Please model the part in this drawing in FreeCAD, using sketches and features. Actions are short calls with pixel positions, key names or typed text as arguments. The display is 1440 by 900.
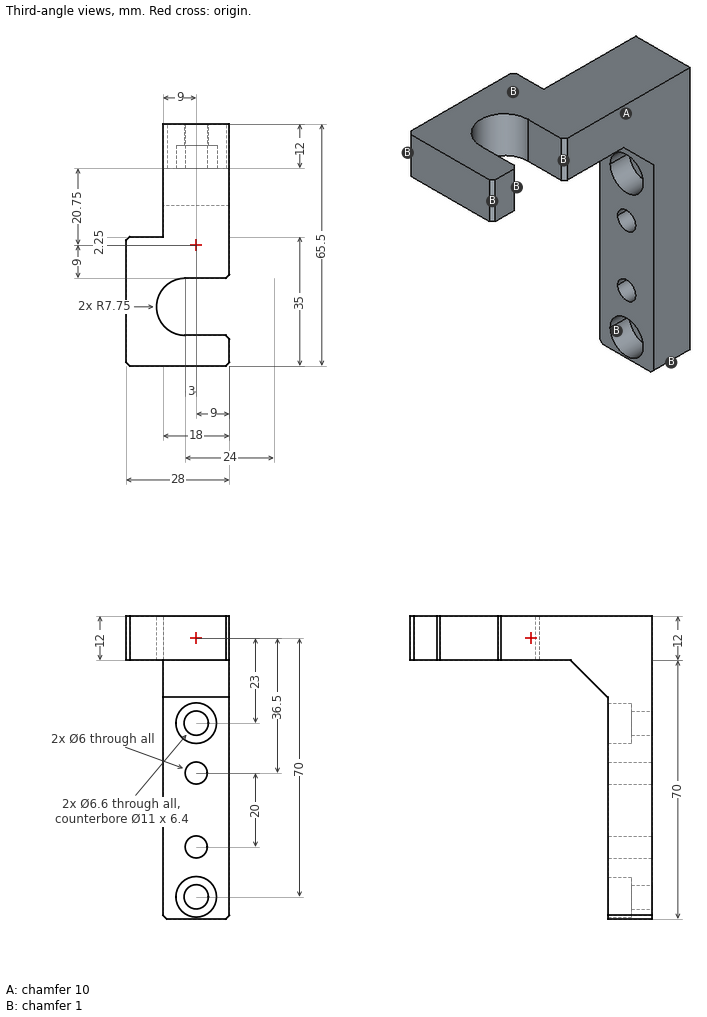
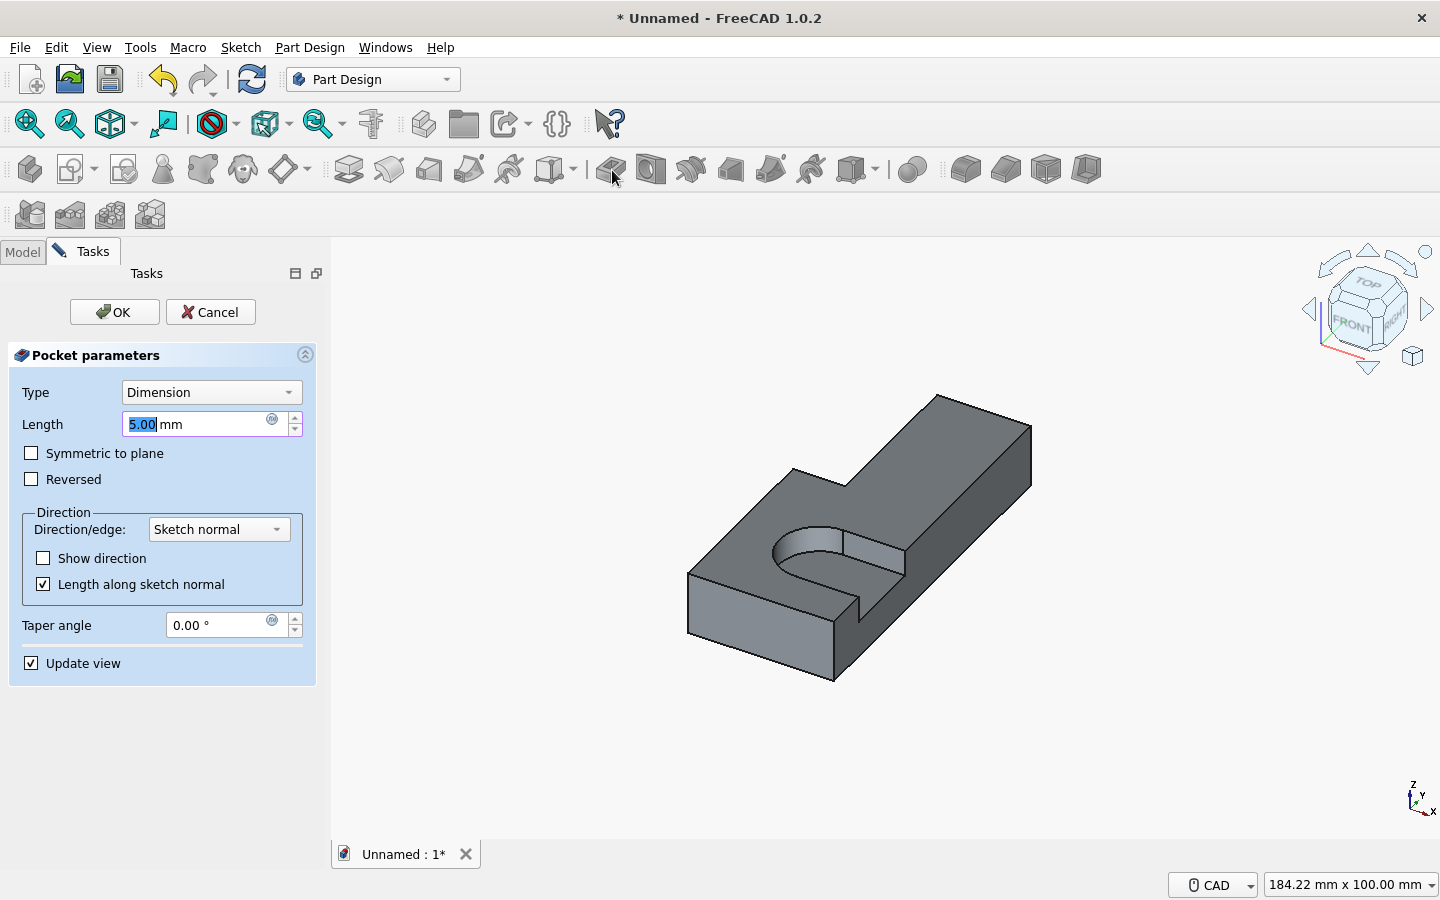
click(212, 392)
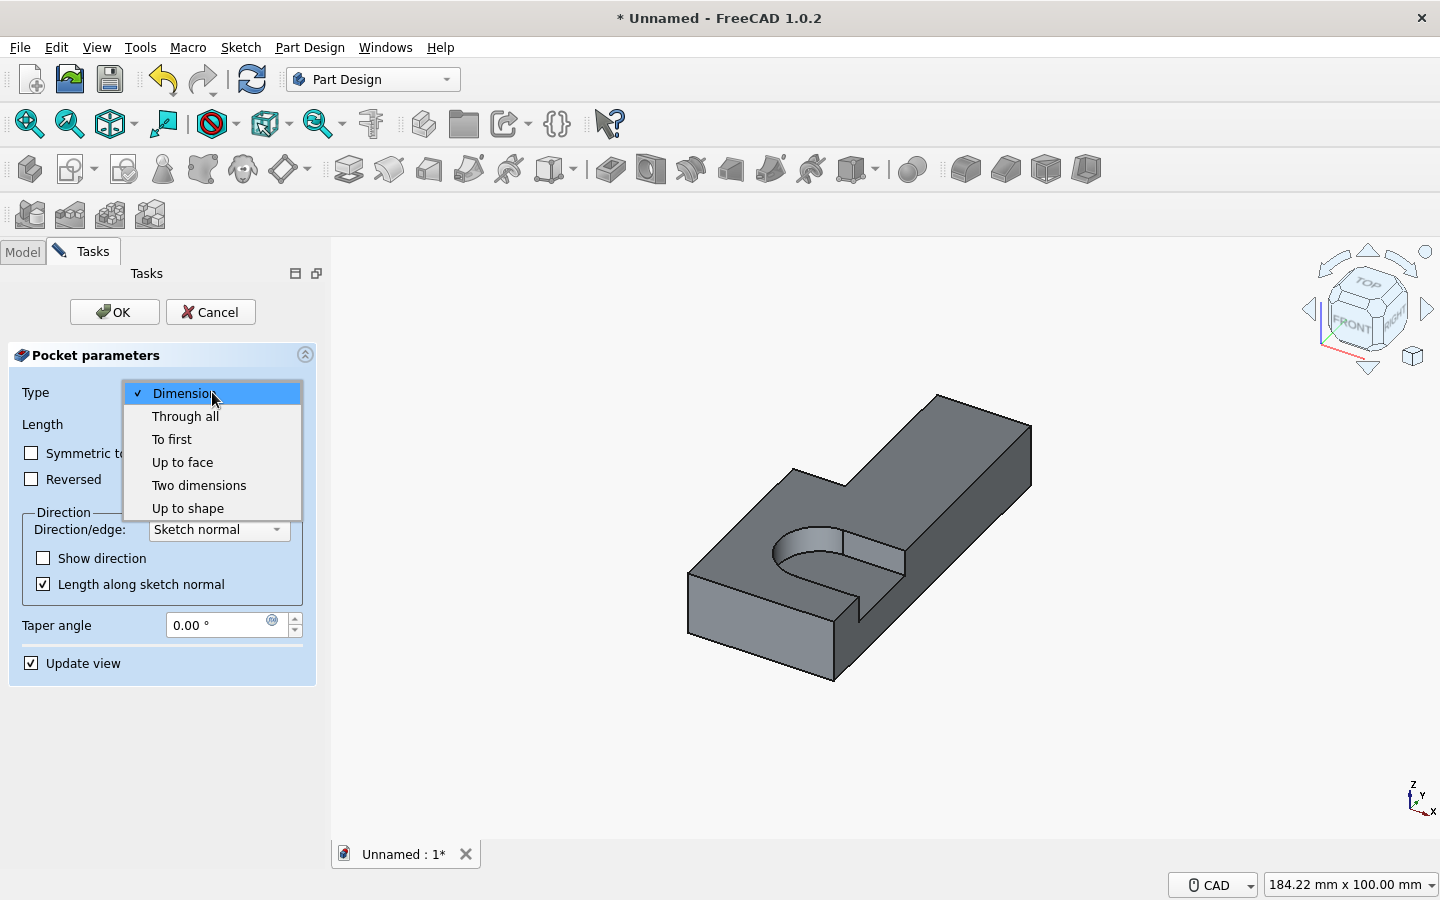
click(212, 416)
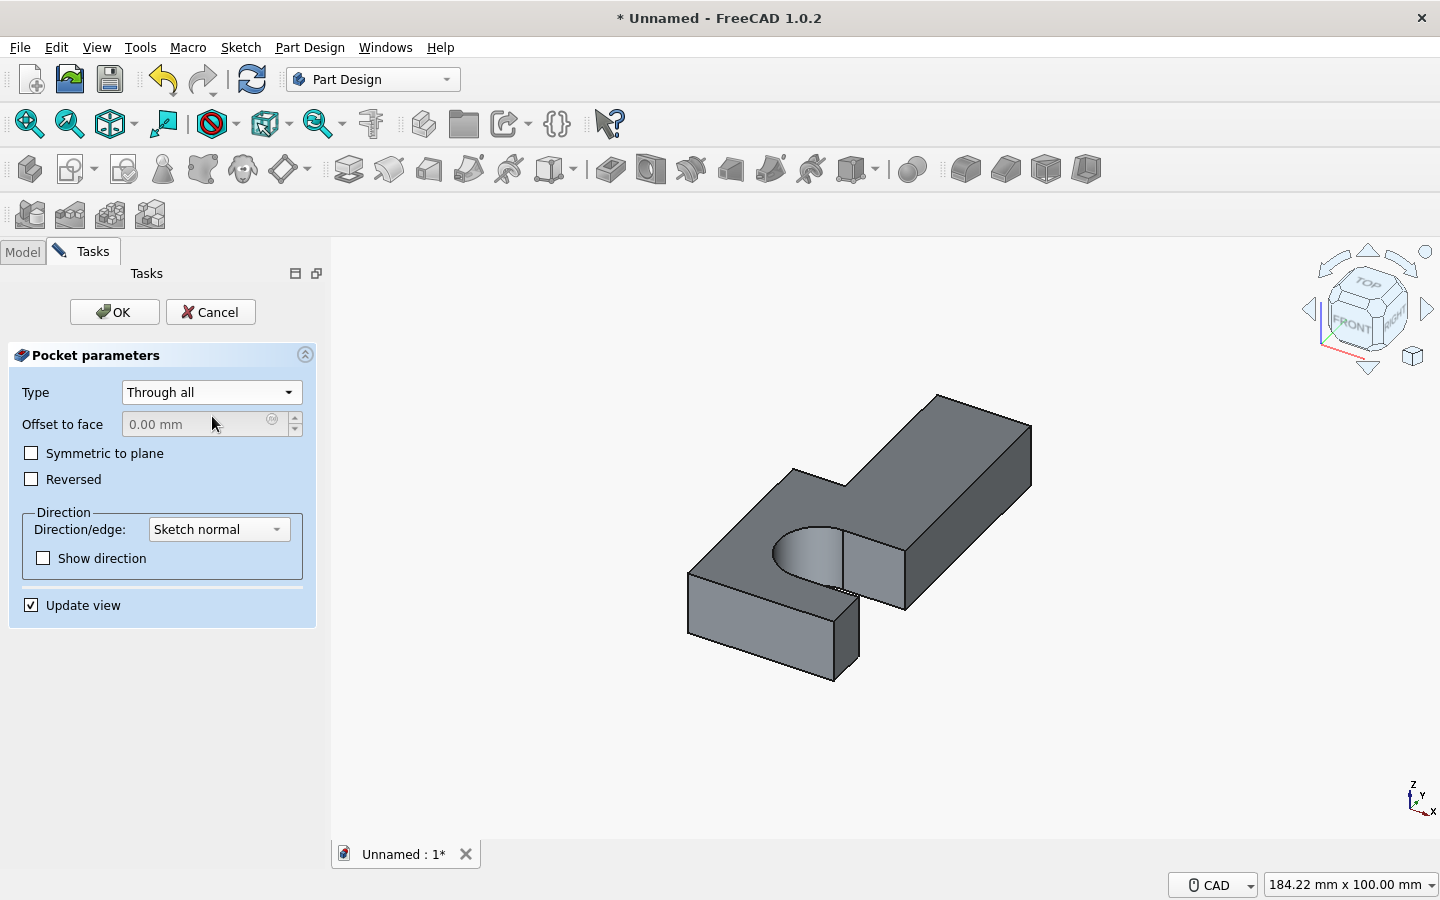
click(115, 312)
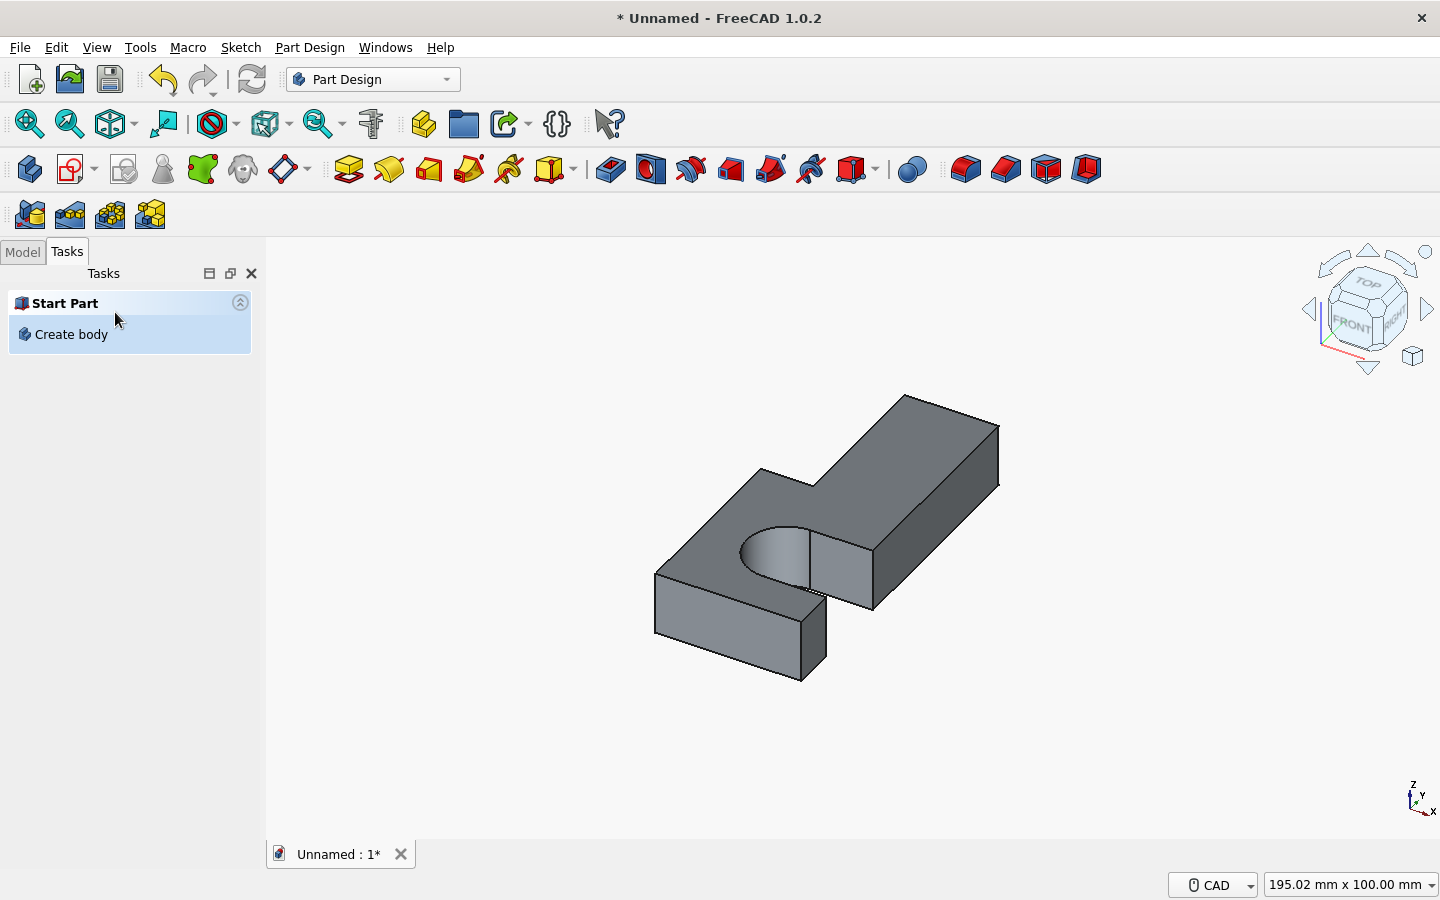
key(5)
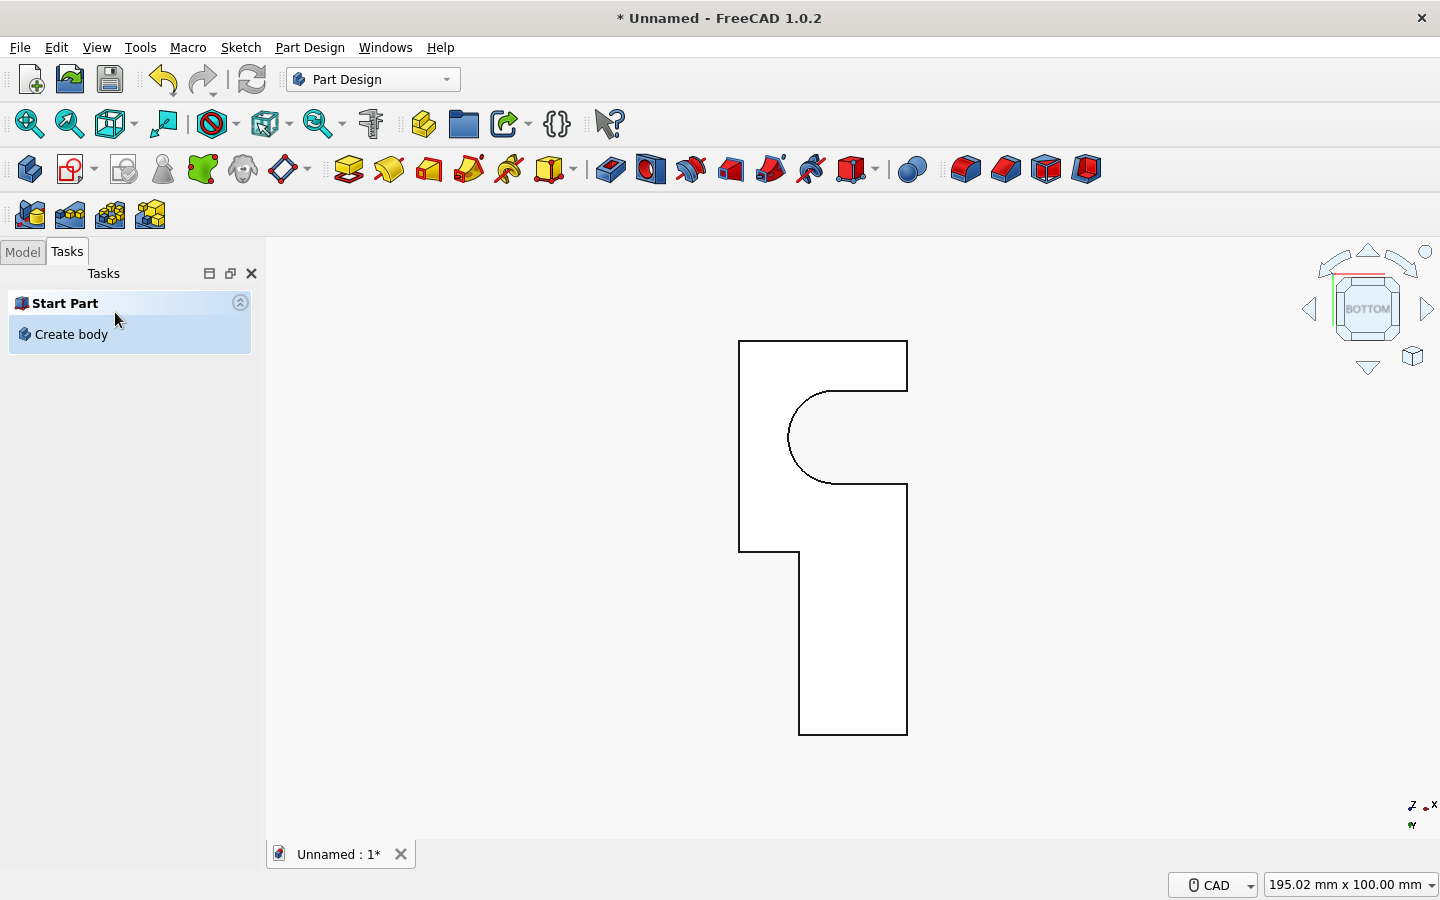
click(847, 537)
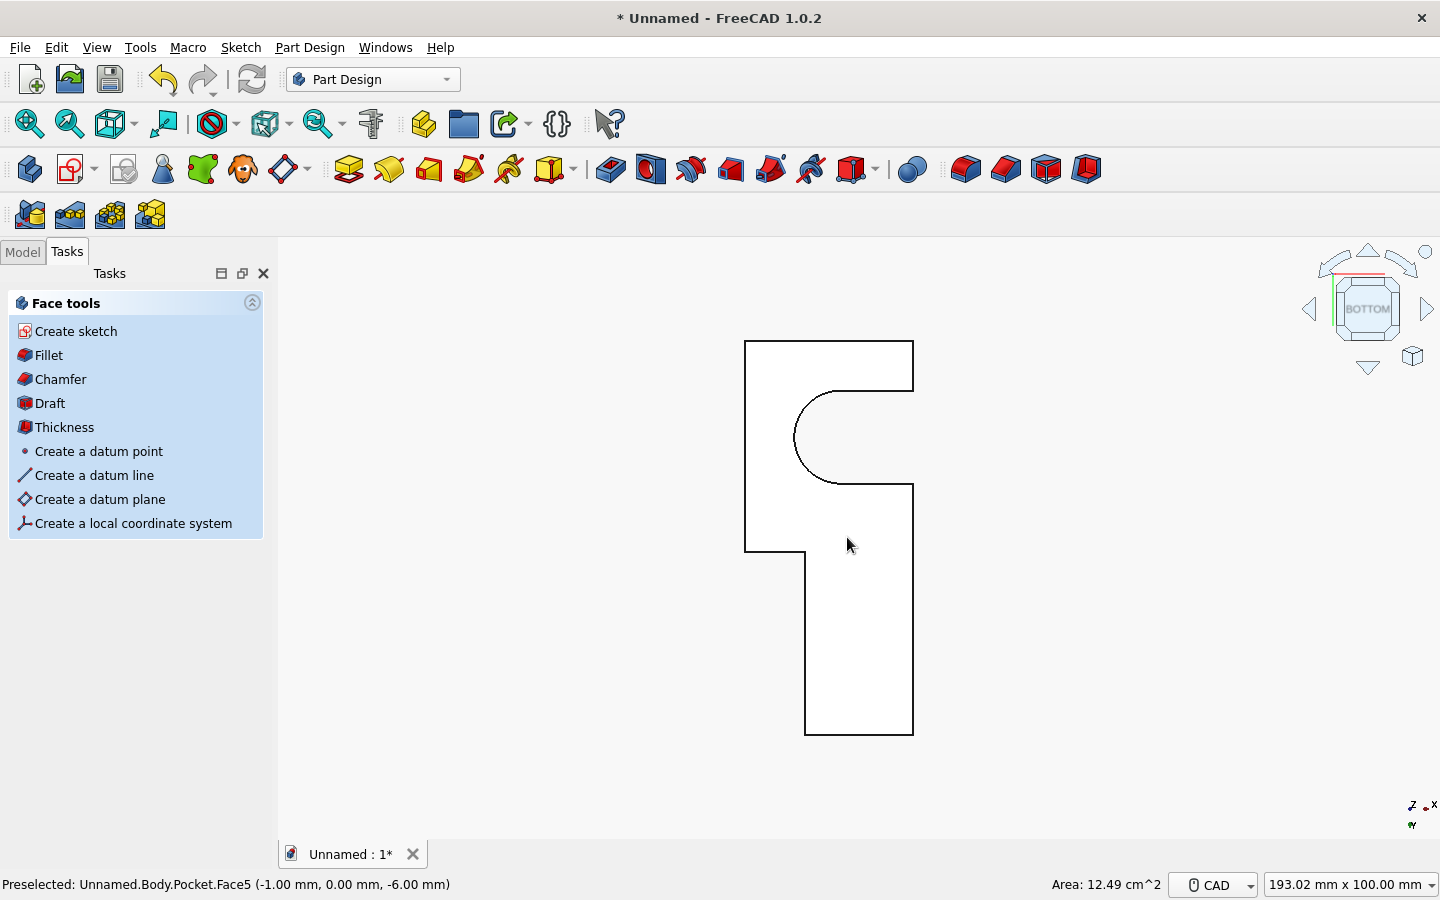
click(70, 170)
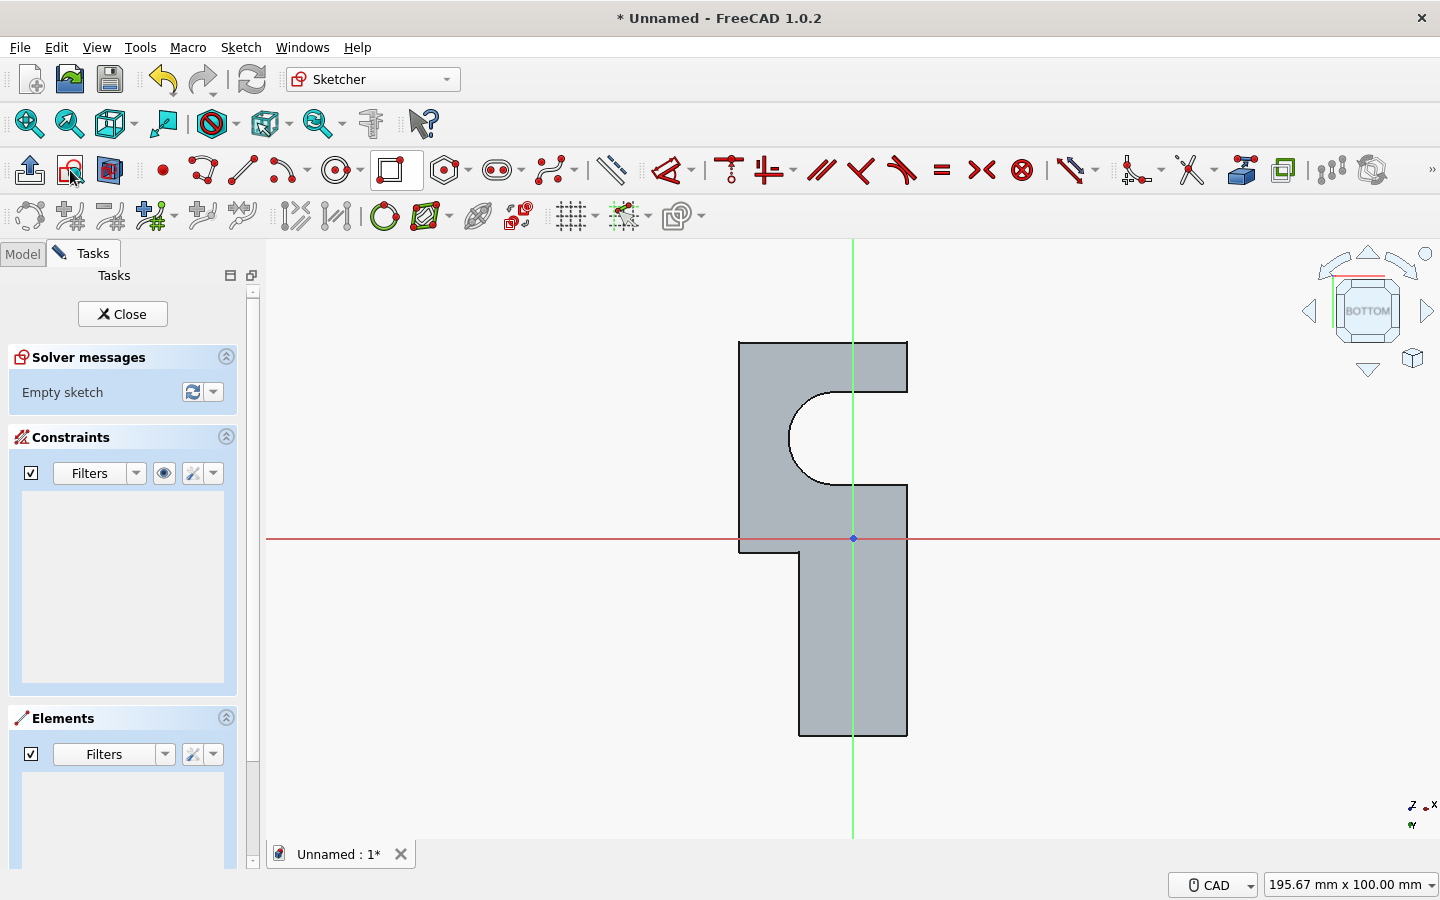
scroll(936, 757, up, 3)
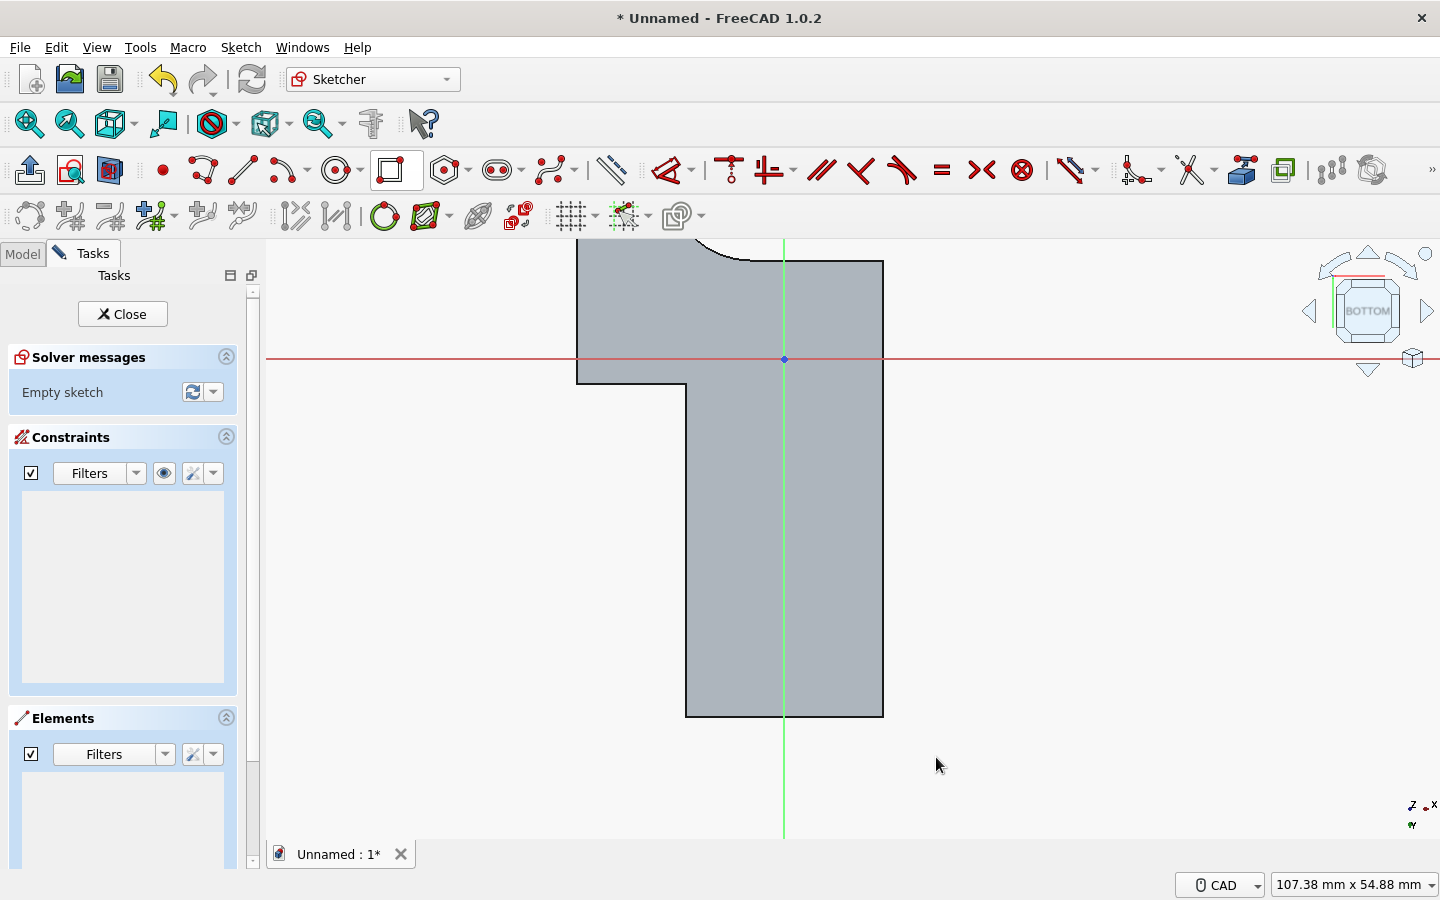
click(390, 170)